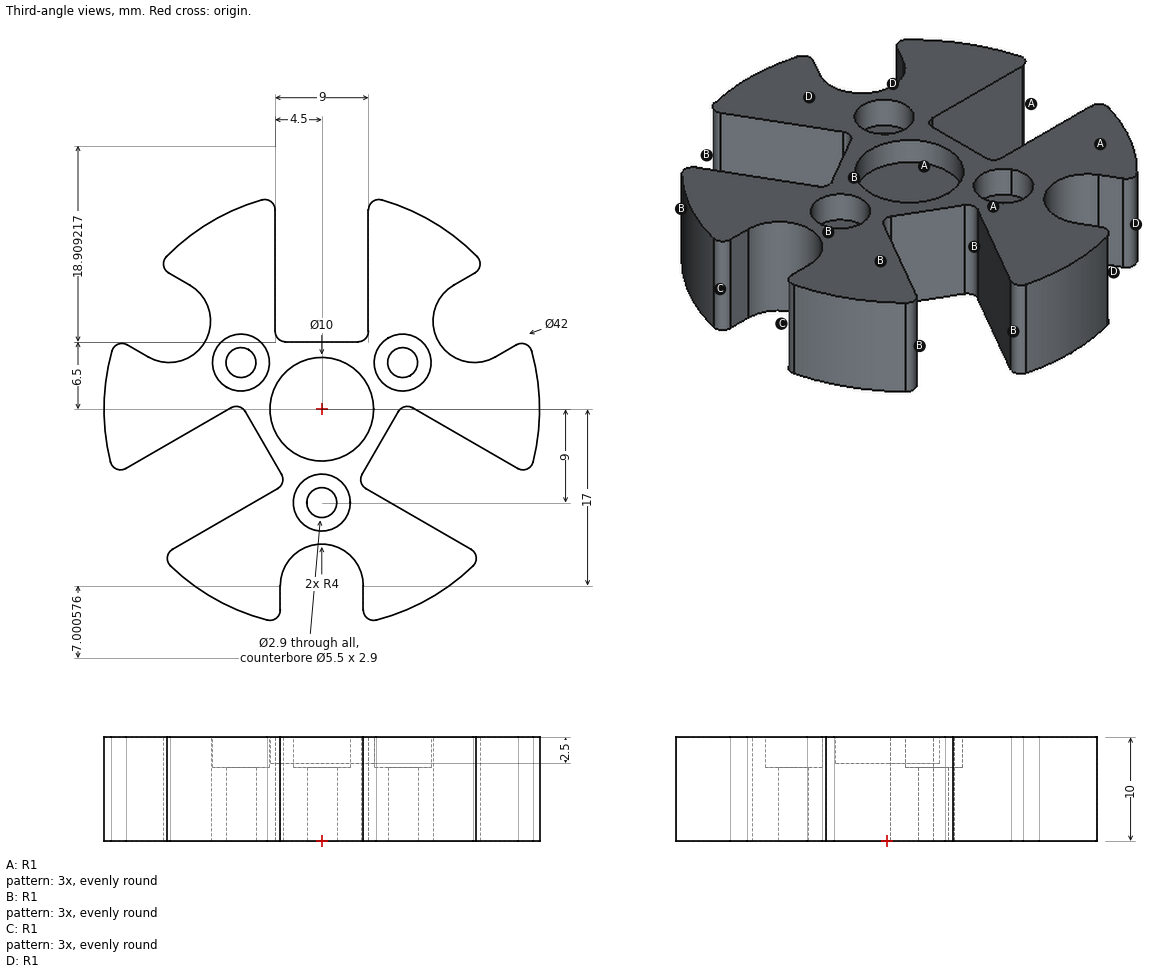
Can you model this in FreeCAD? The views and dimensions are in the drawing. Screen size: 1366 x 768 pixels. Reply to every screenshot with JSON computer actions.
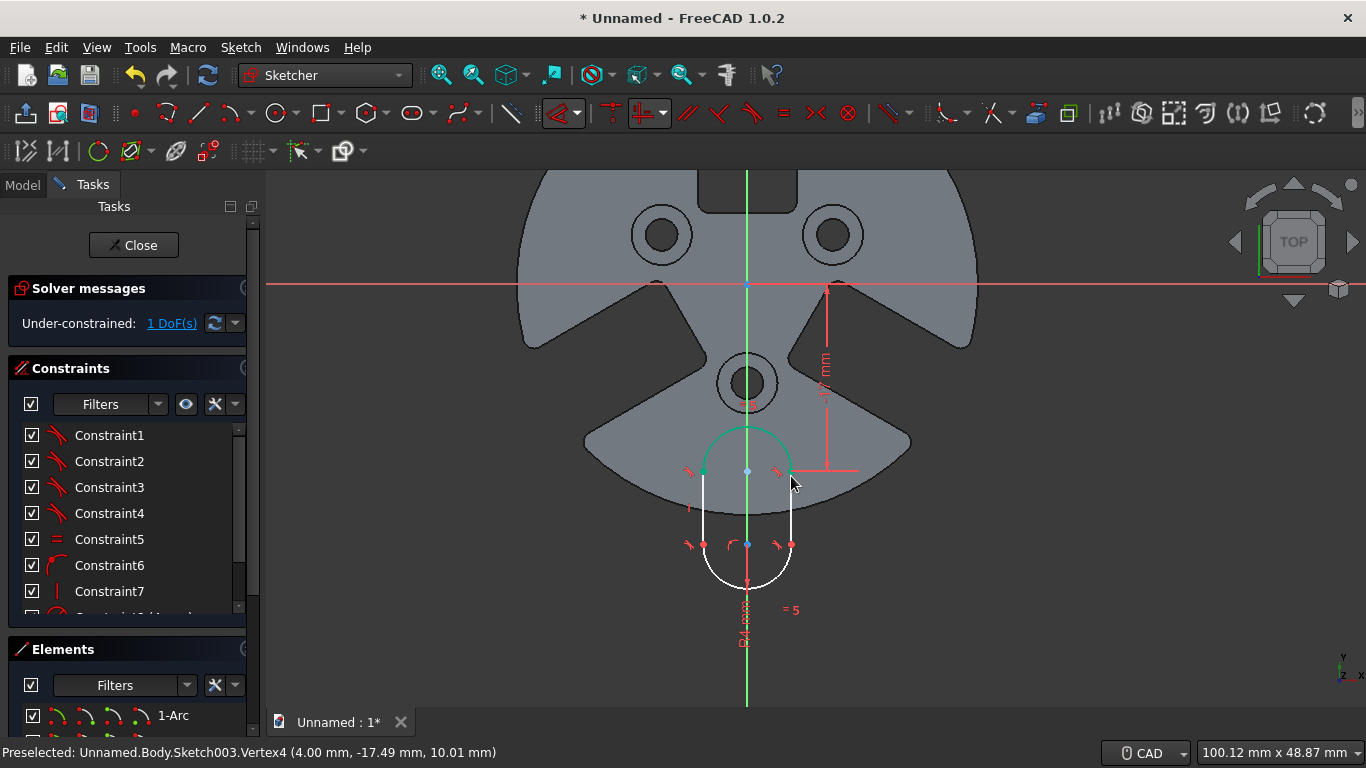
{"action": "left_click", "coordinate": [703, 523]}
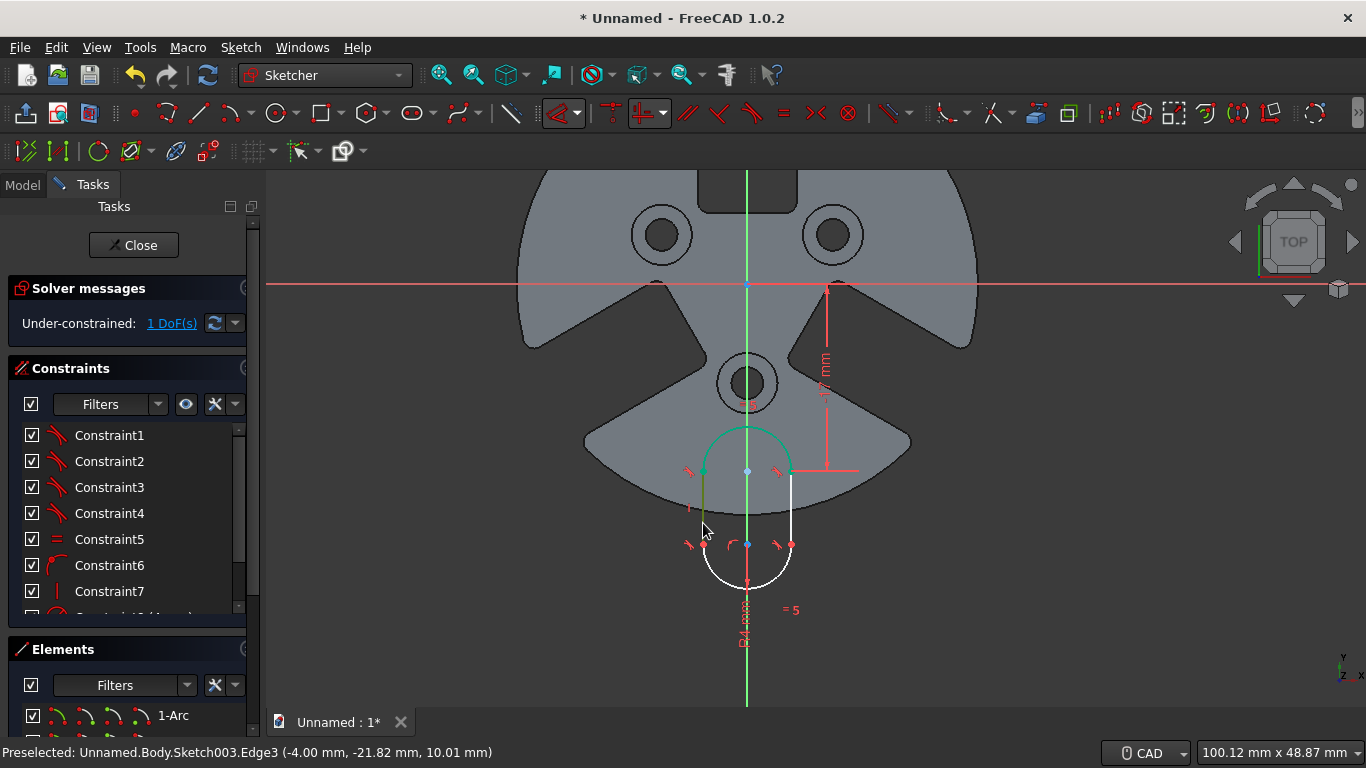
{"action": "key", "text": "i"}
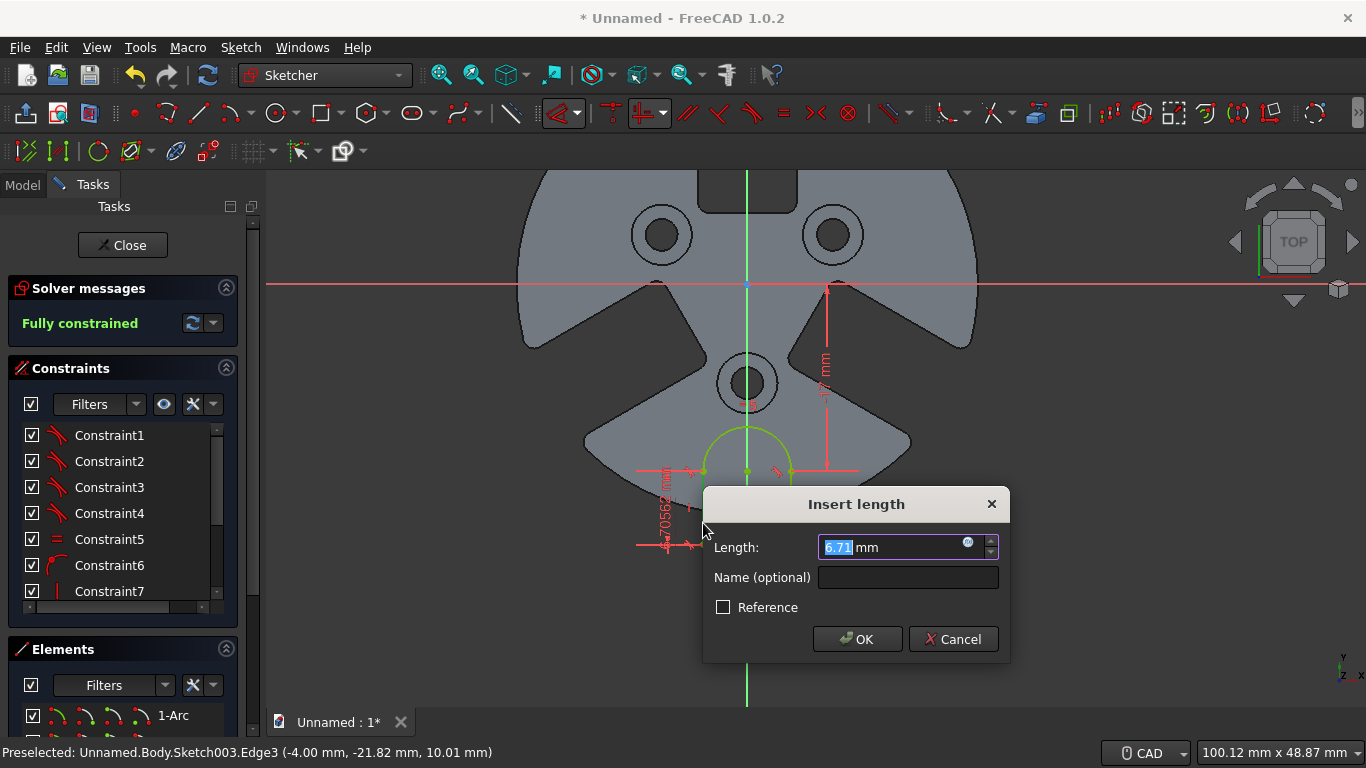
{"action": "type", "text": "7.000576"}
{"action": "key", "text": "Return"}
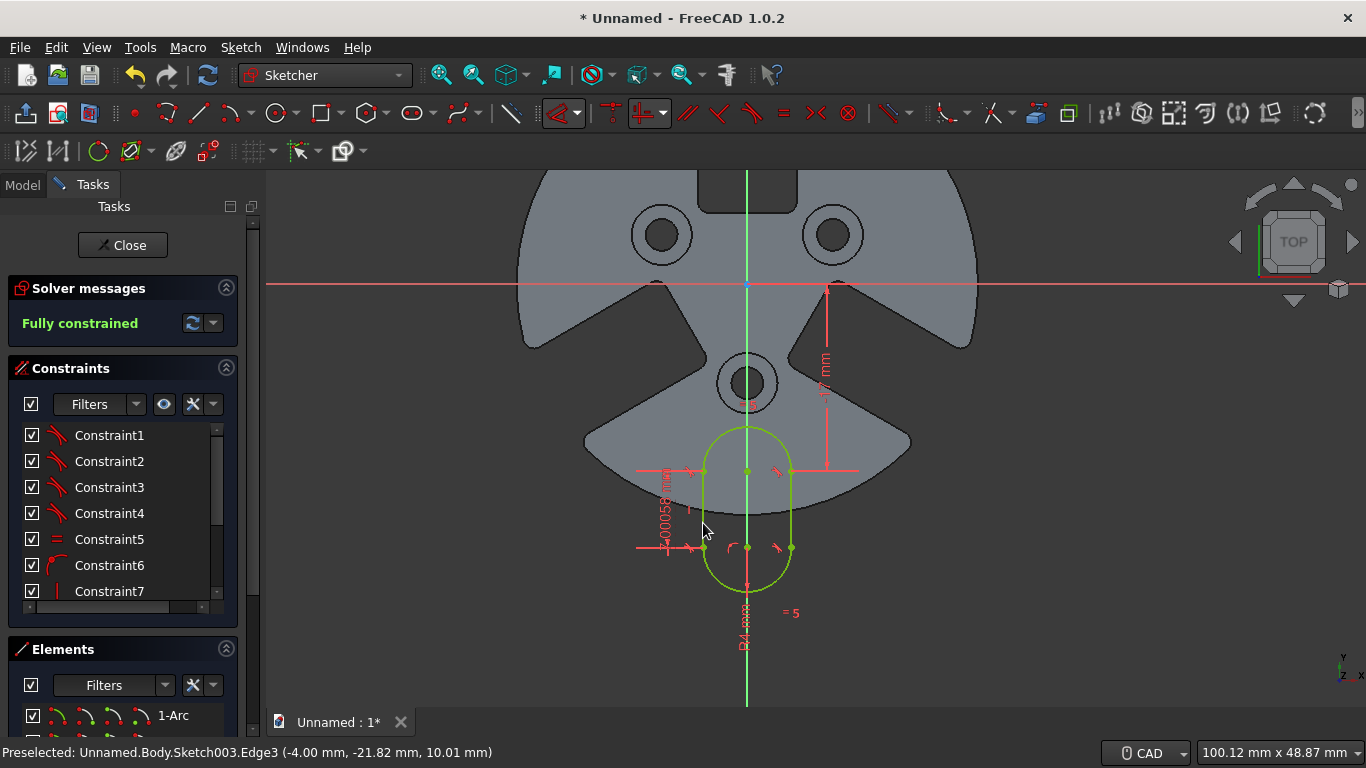
{"action": "left_click", "coordinate": [123, 245]}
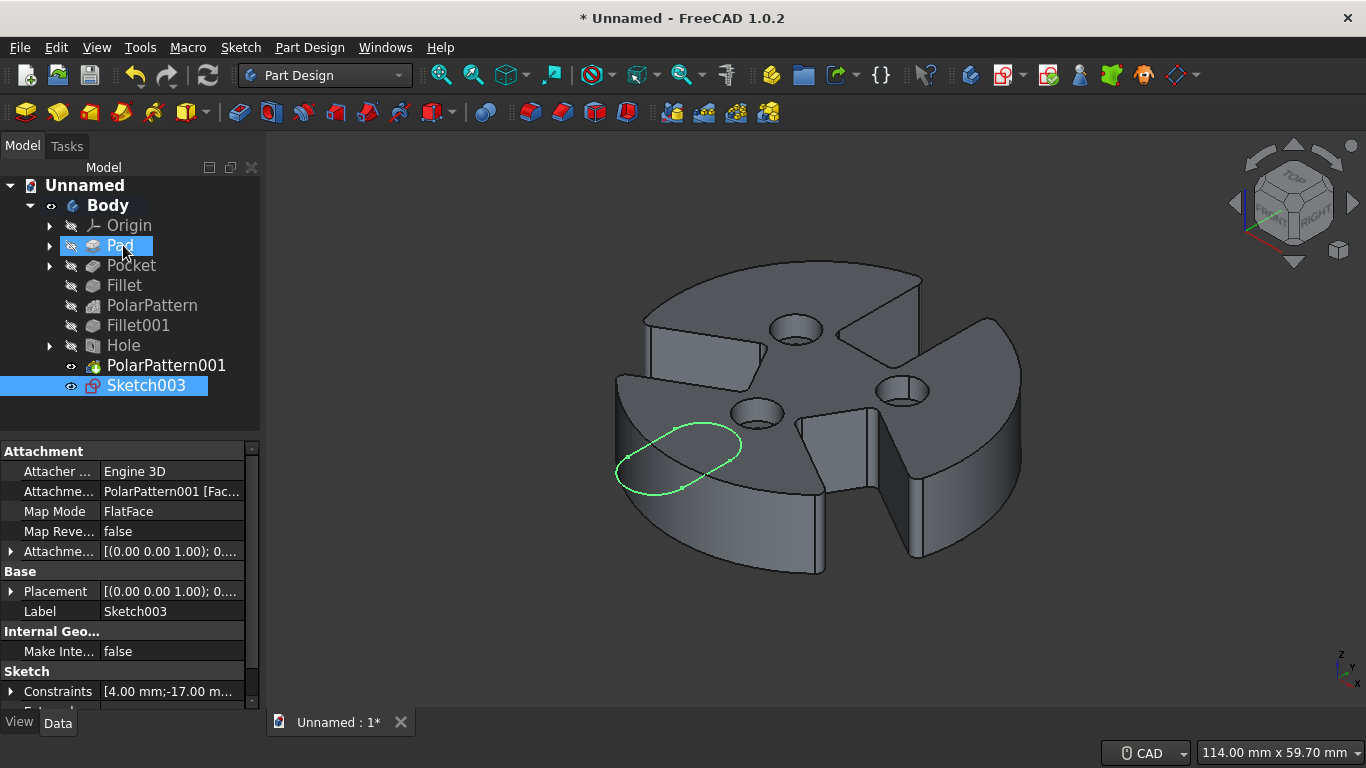
{"action": "left_click", "coordinate": [240, 112]}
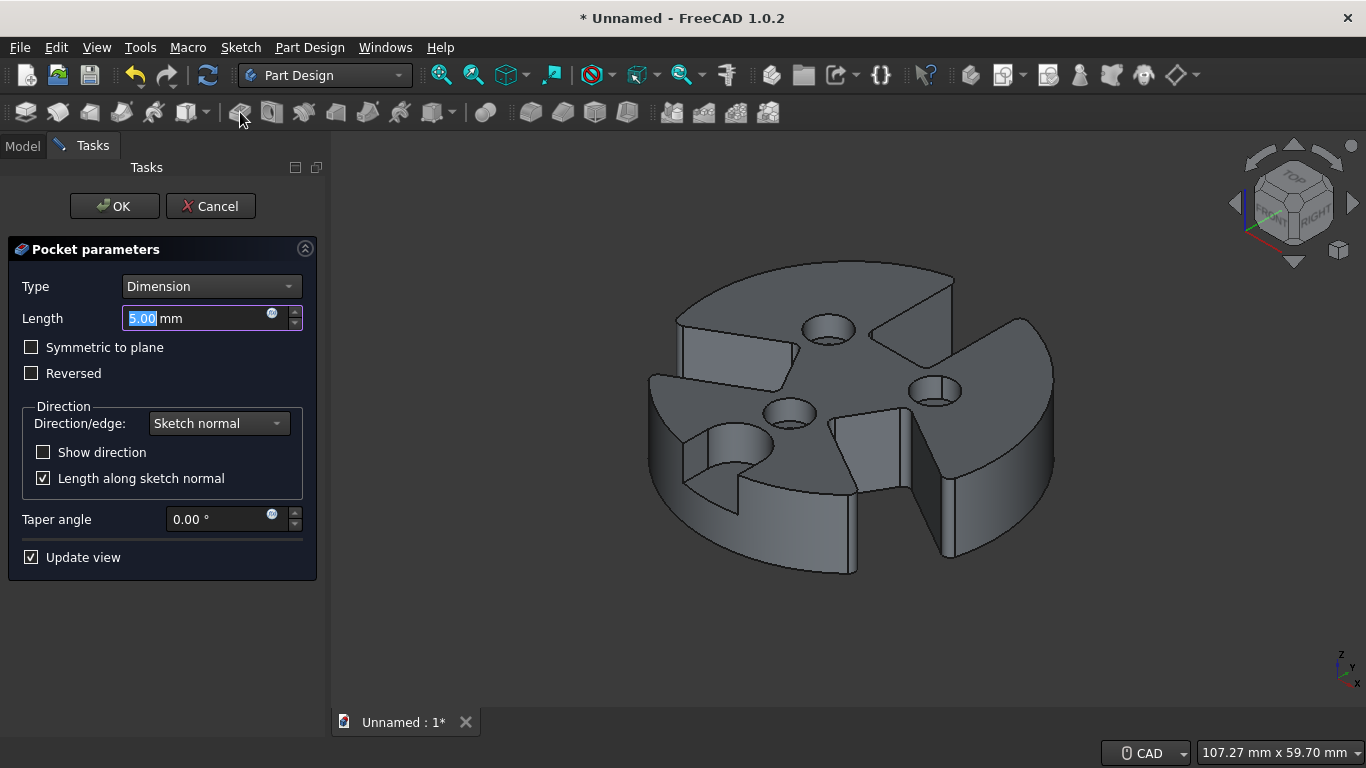
{"action": "left_click", "coordinate": [212, 286]}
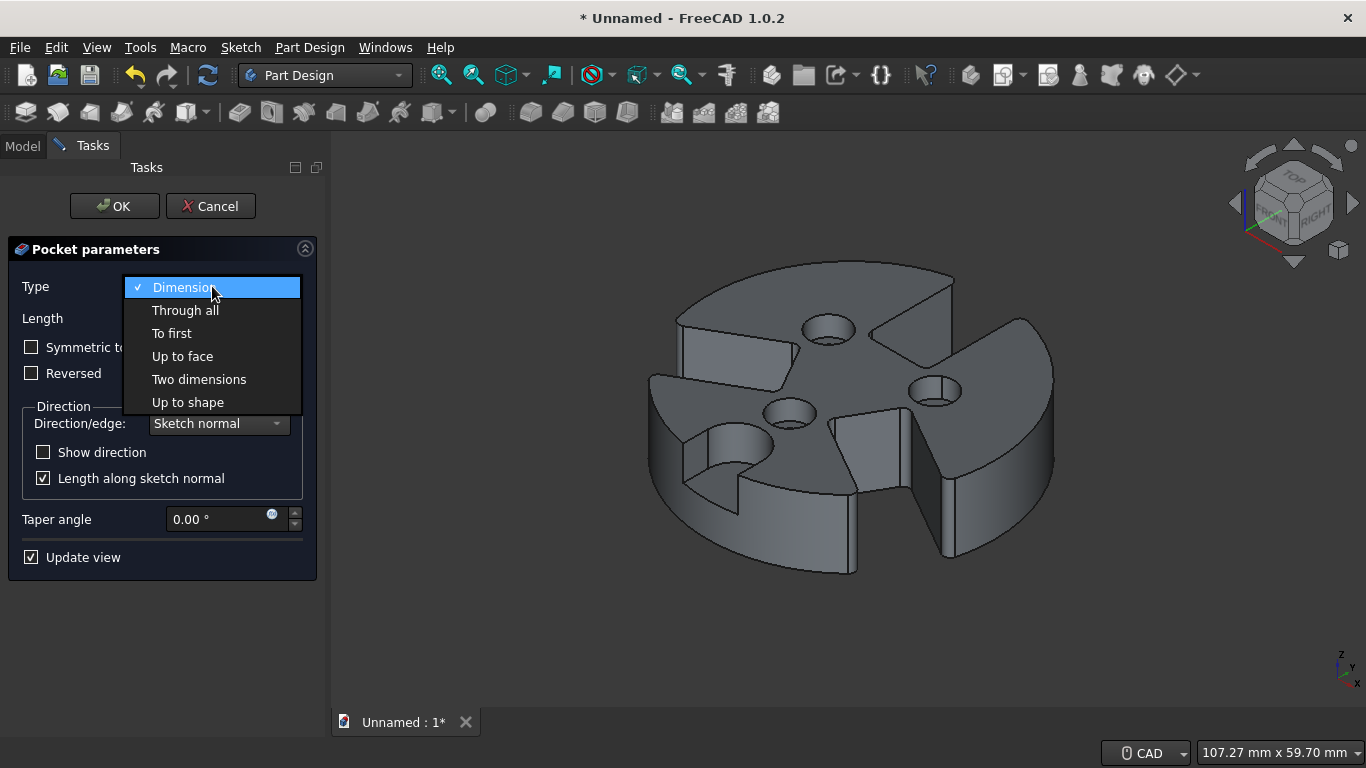
{"action": "left_click", "coordinate": [212, 310]}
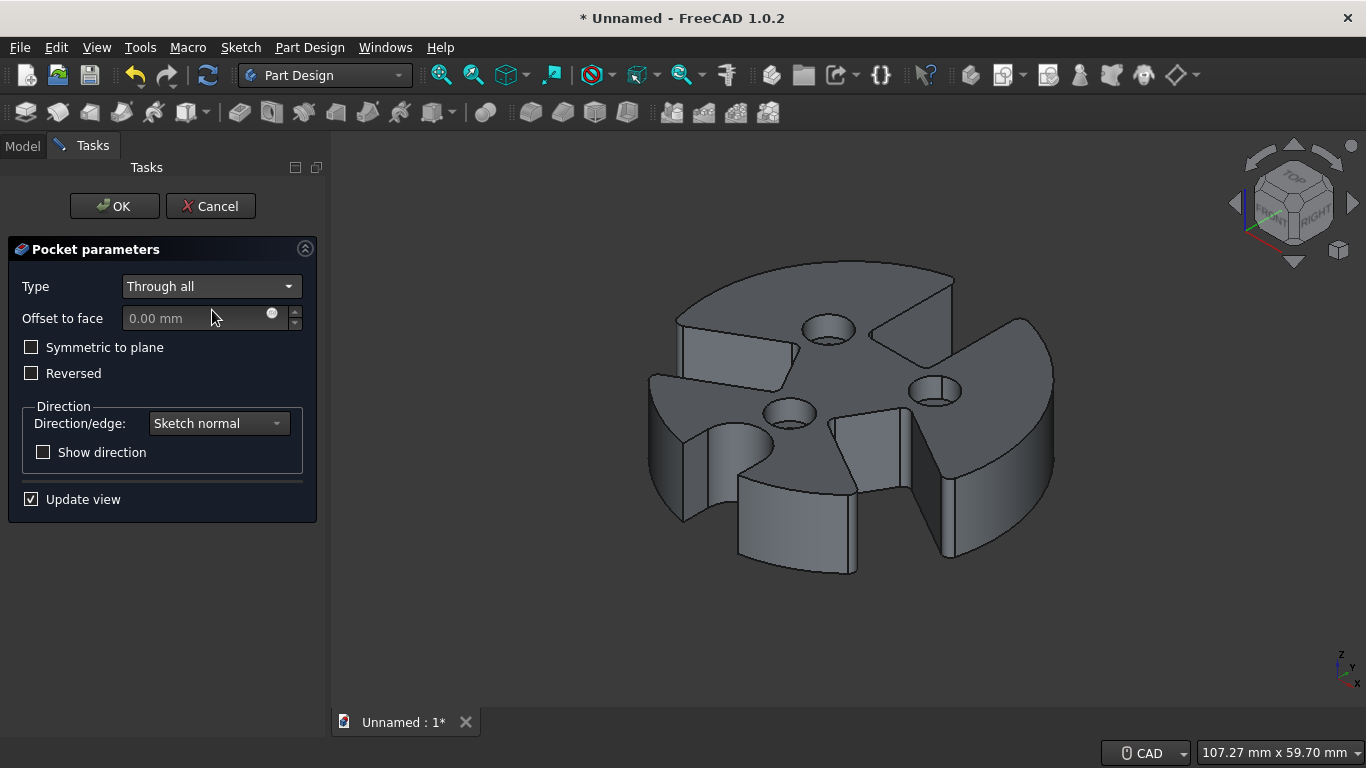
{"action": "left_click", "coordinate": [115, 206]}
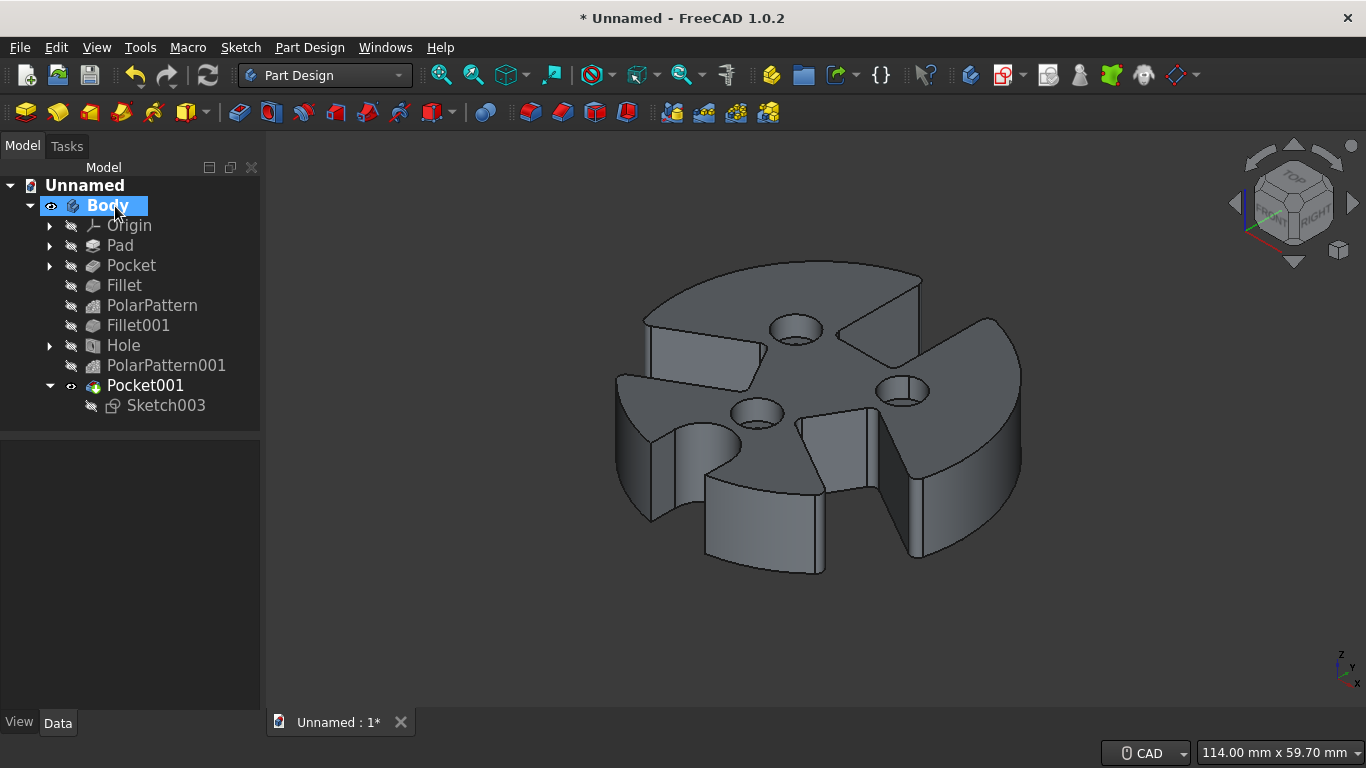
{"action": "left_click", "coordinate": [651, 482]}